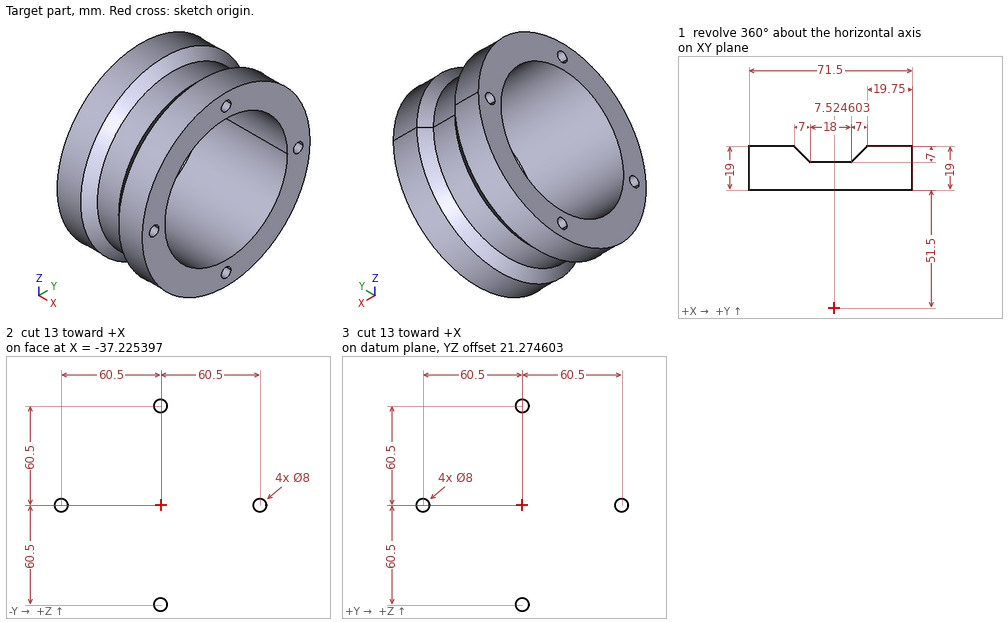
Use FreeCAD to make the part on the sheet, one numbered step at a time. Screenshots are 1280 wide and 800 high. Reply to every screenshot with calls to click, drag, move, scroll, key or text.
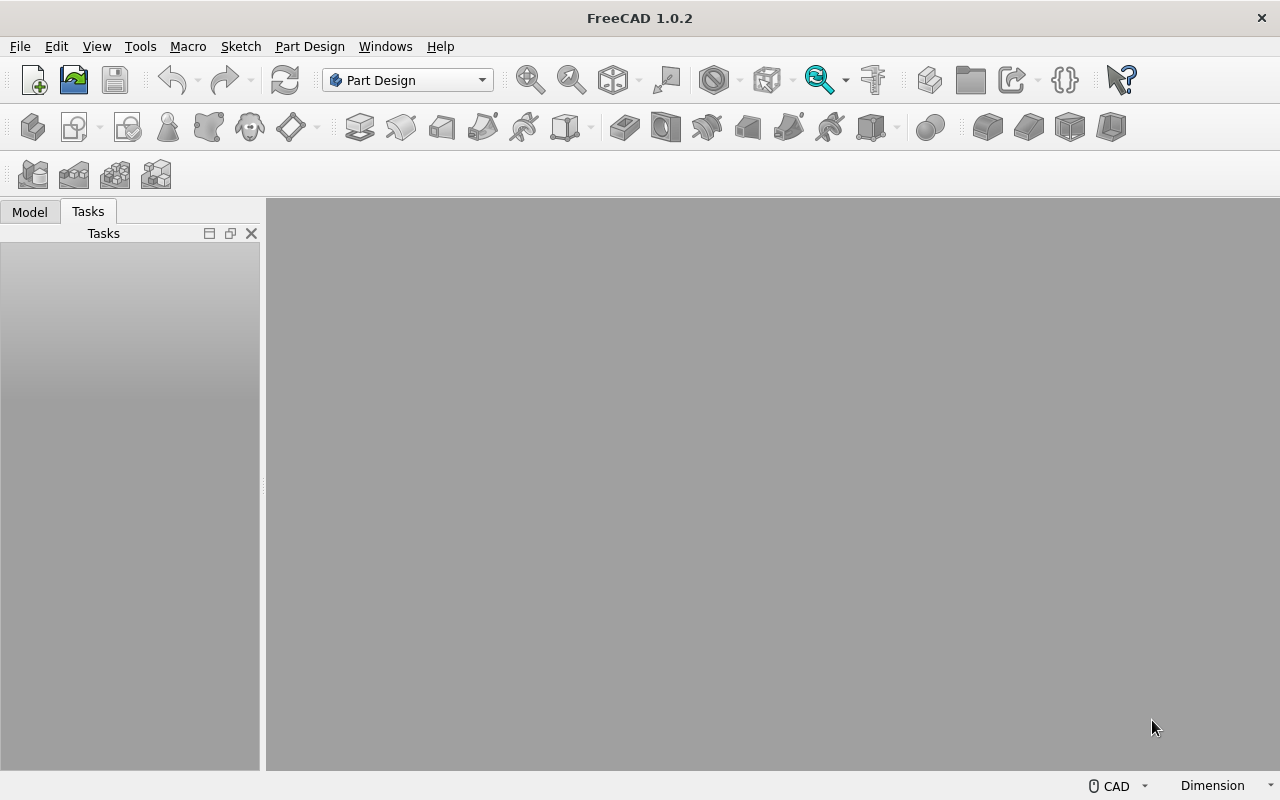
click(33, 80)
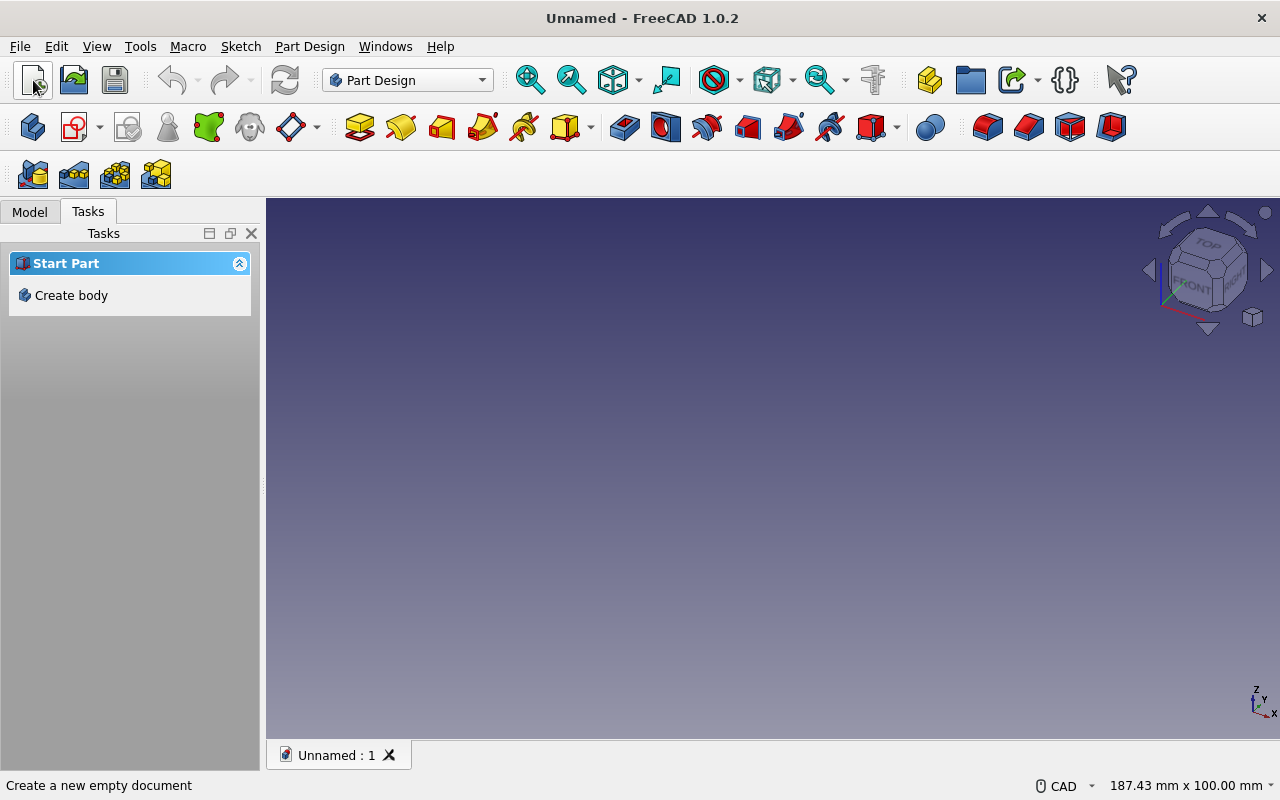
click(74, 128)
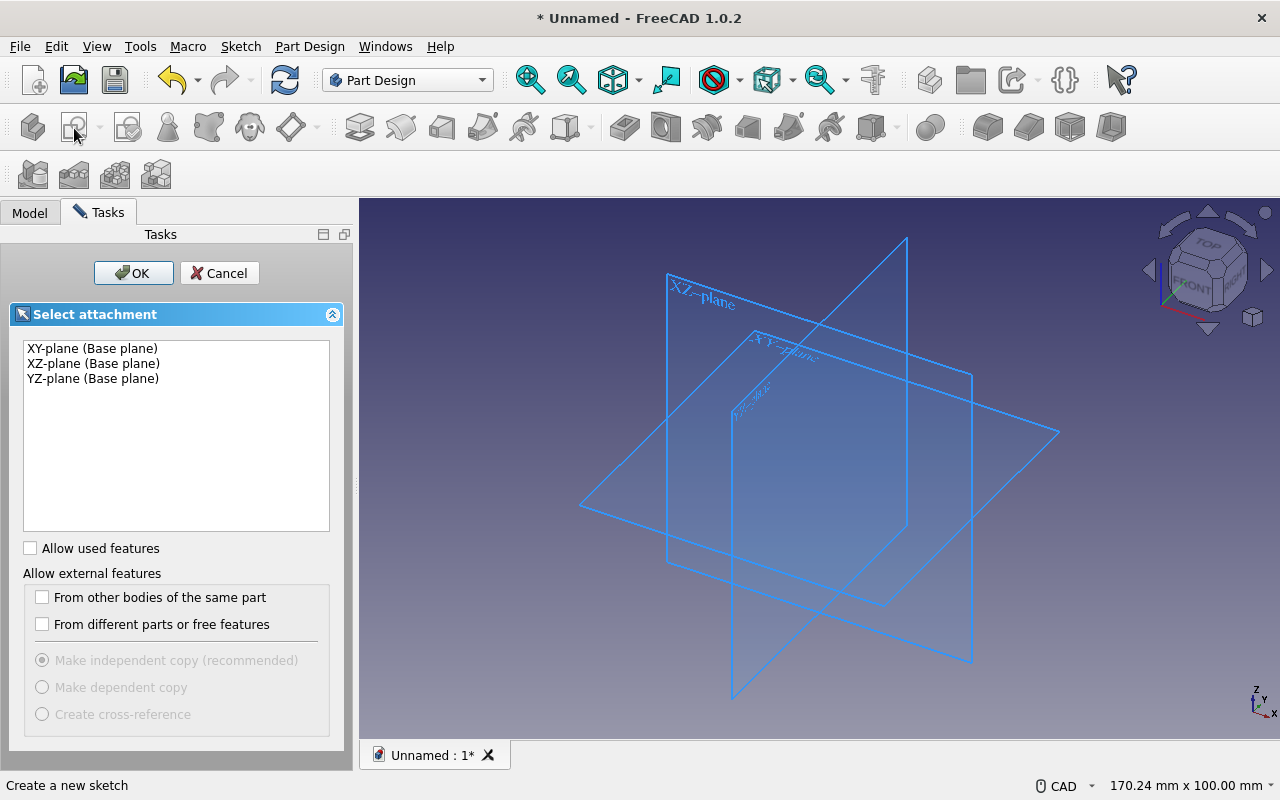
click(84, 348)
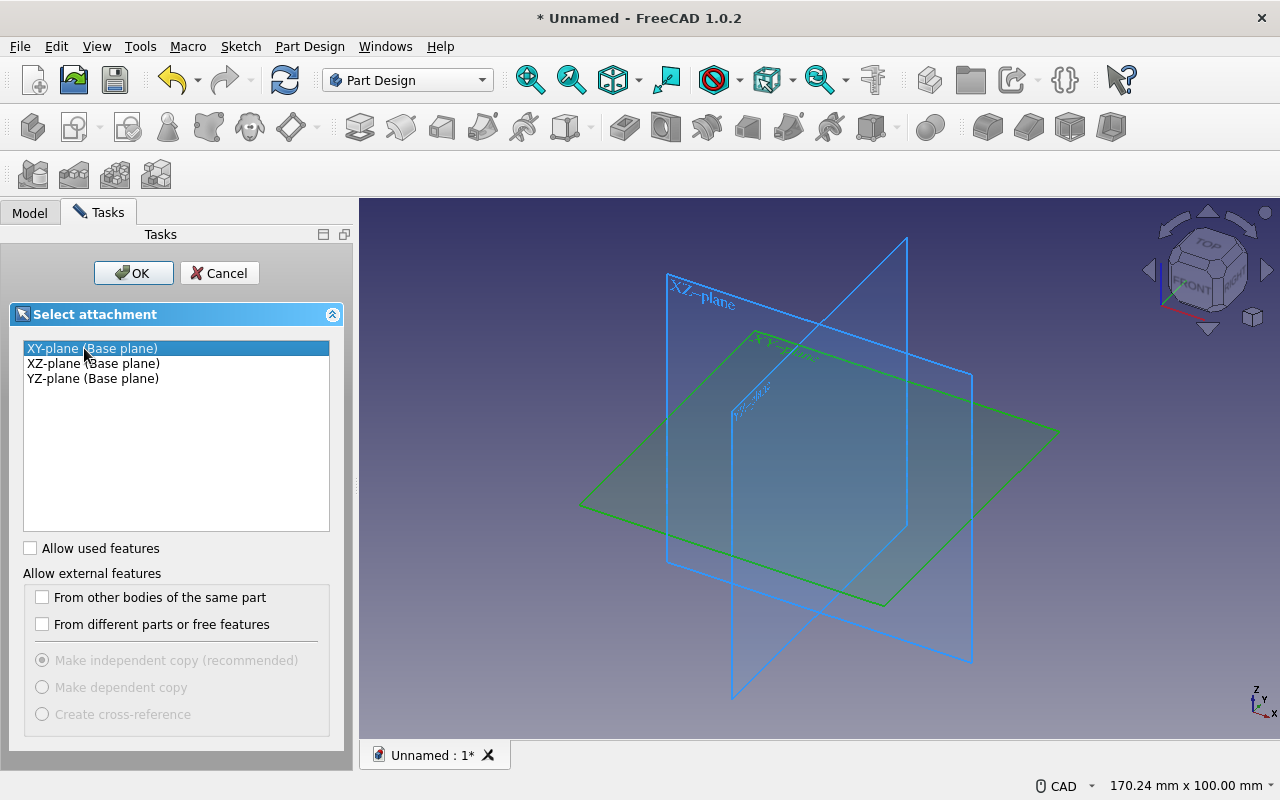
click(134, 273)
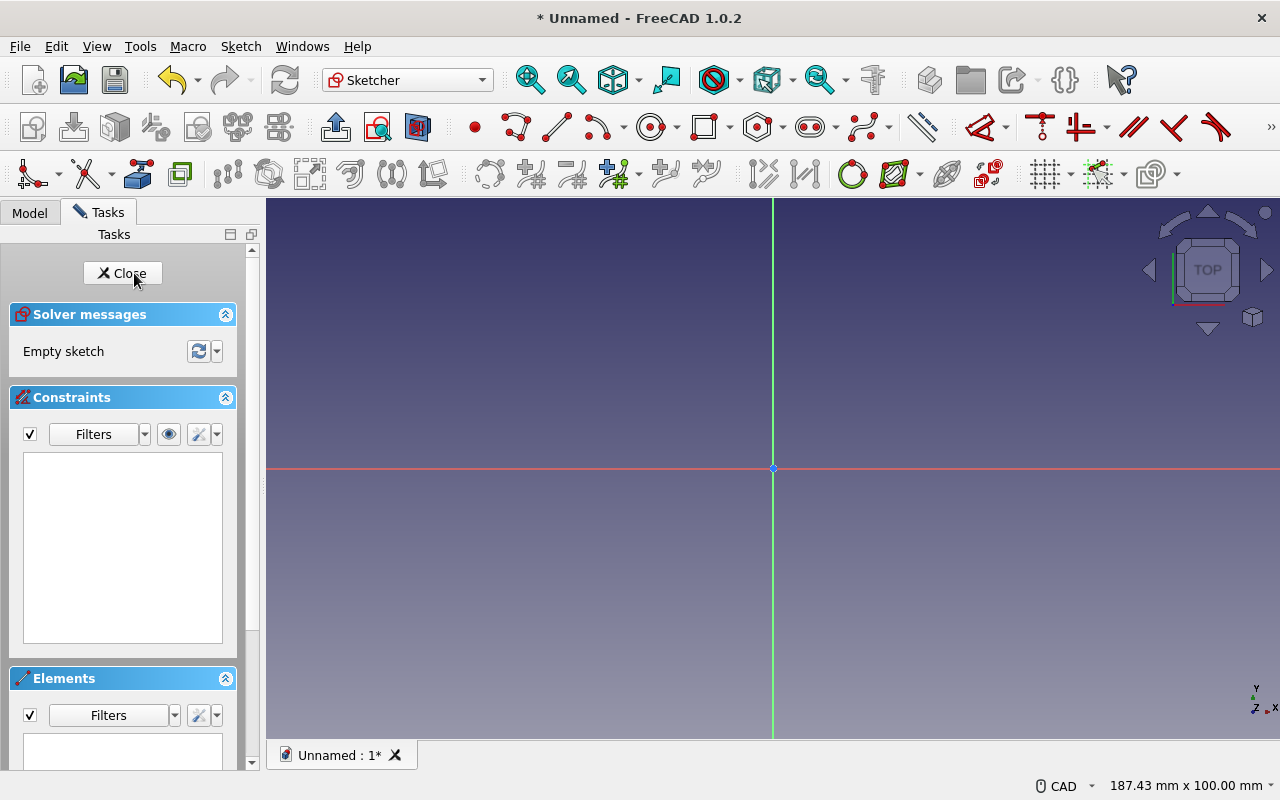
scroll(581, 711, down, 2)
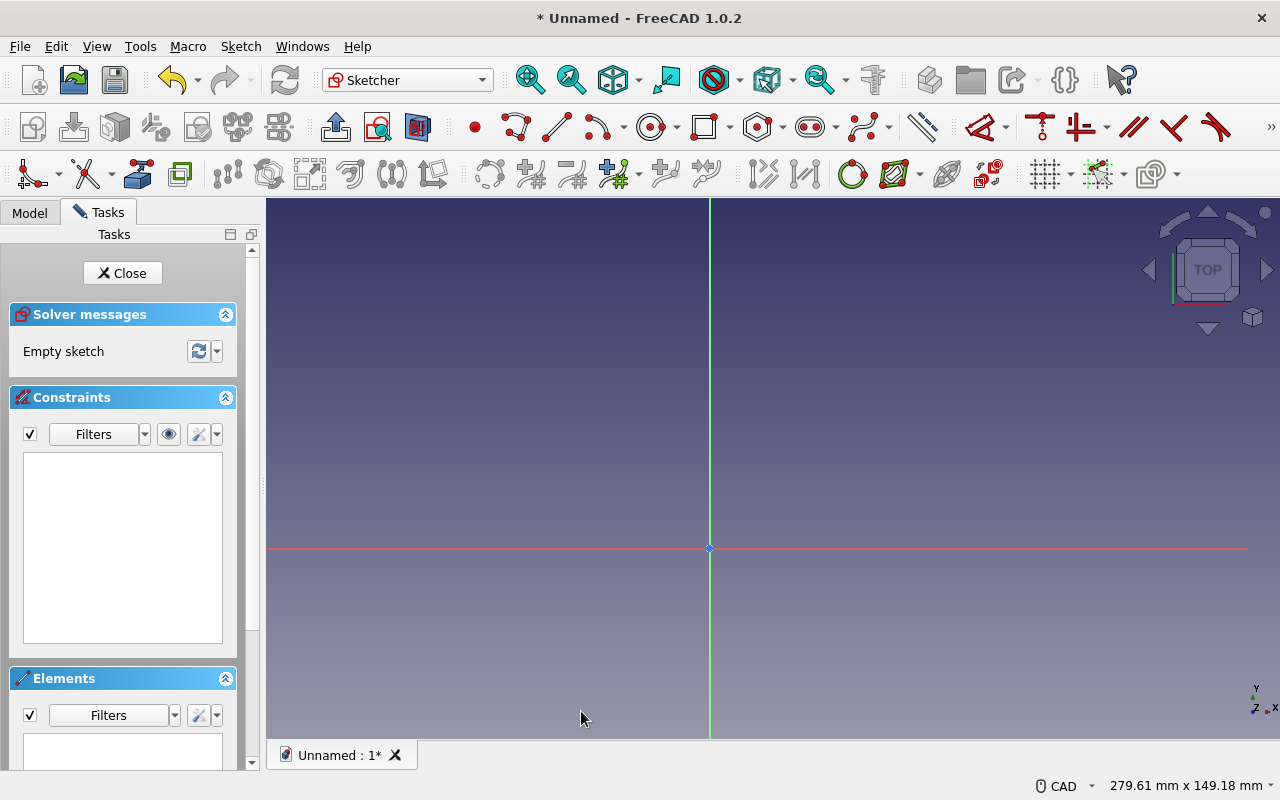
click(516, 128)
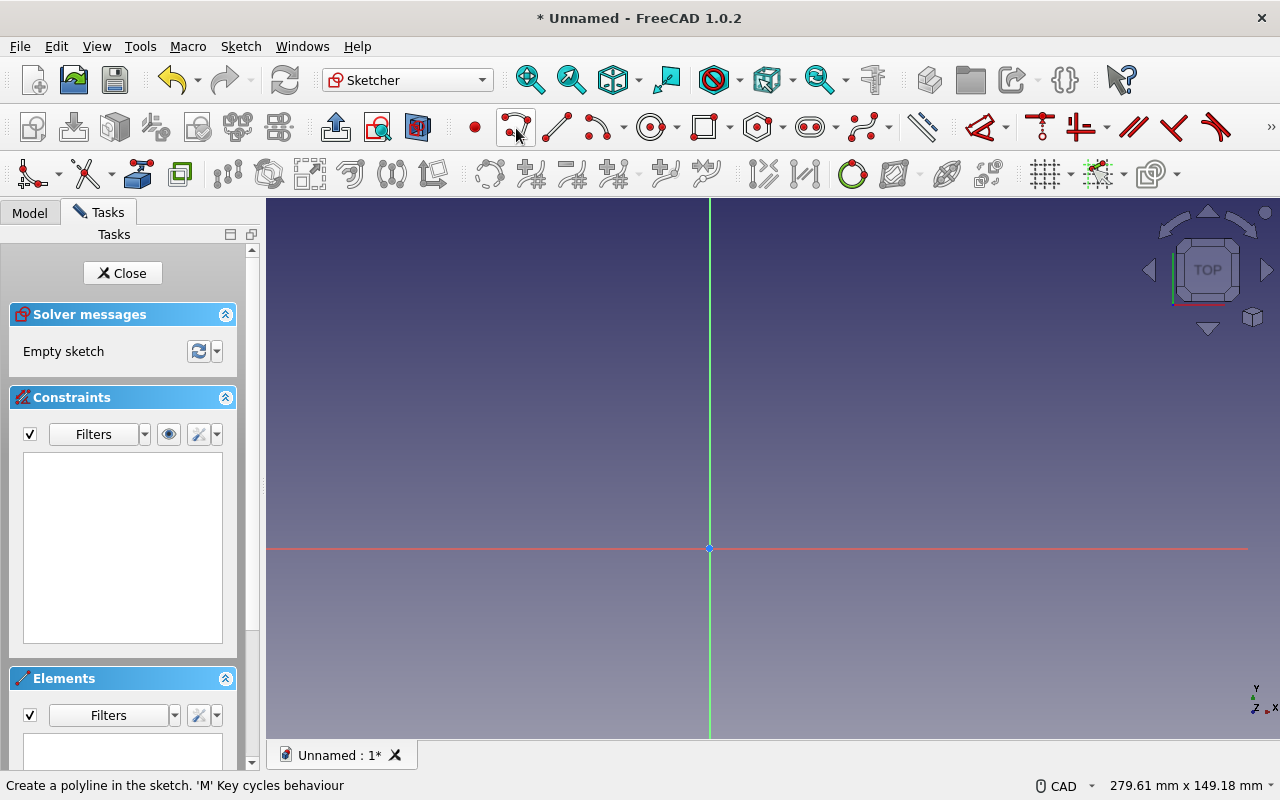
click(834, 362)
click(834, 293)
click(762, 293)
click(737, 318)
click(672, 318)
click(646, 293)
click(575, 293)
click(575, 362)
click(834, 363)
key(Escape)
key(Escape)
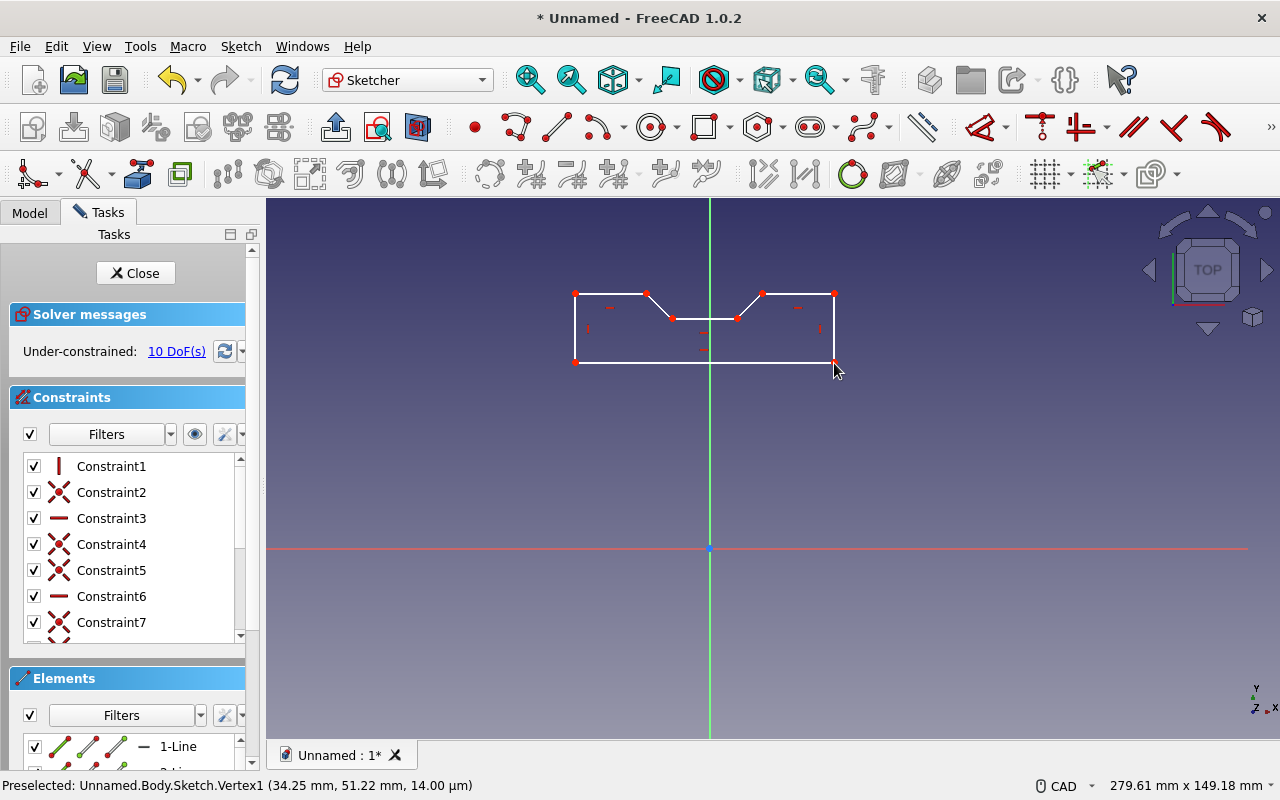
click(980, 128)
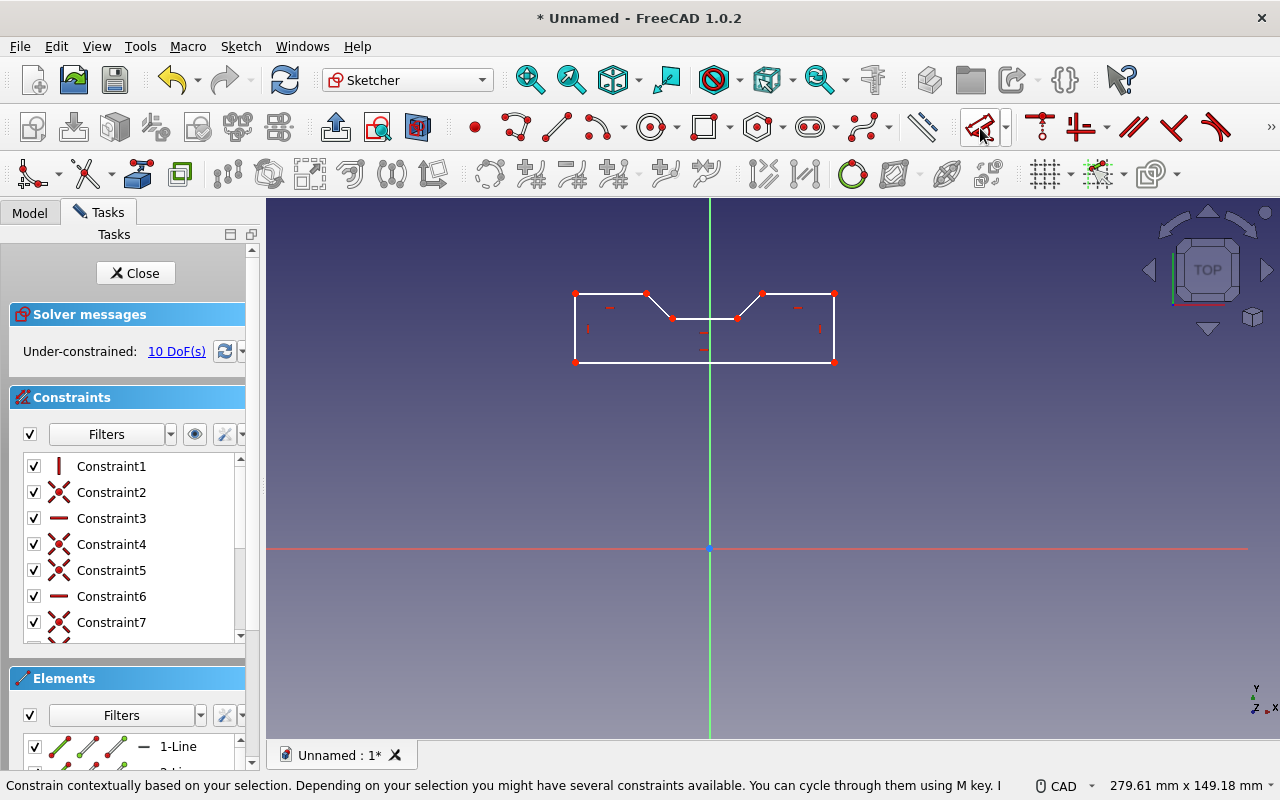
click(834, 342)
click(868, 328)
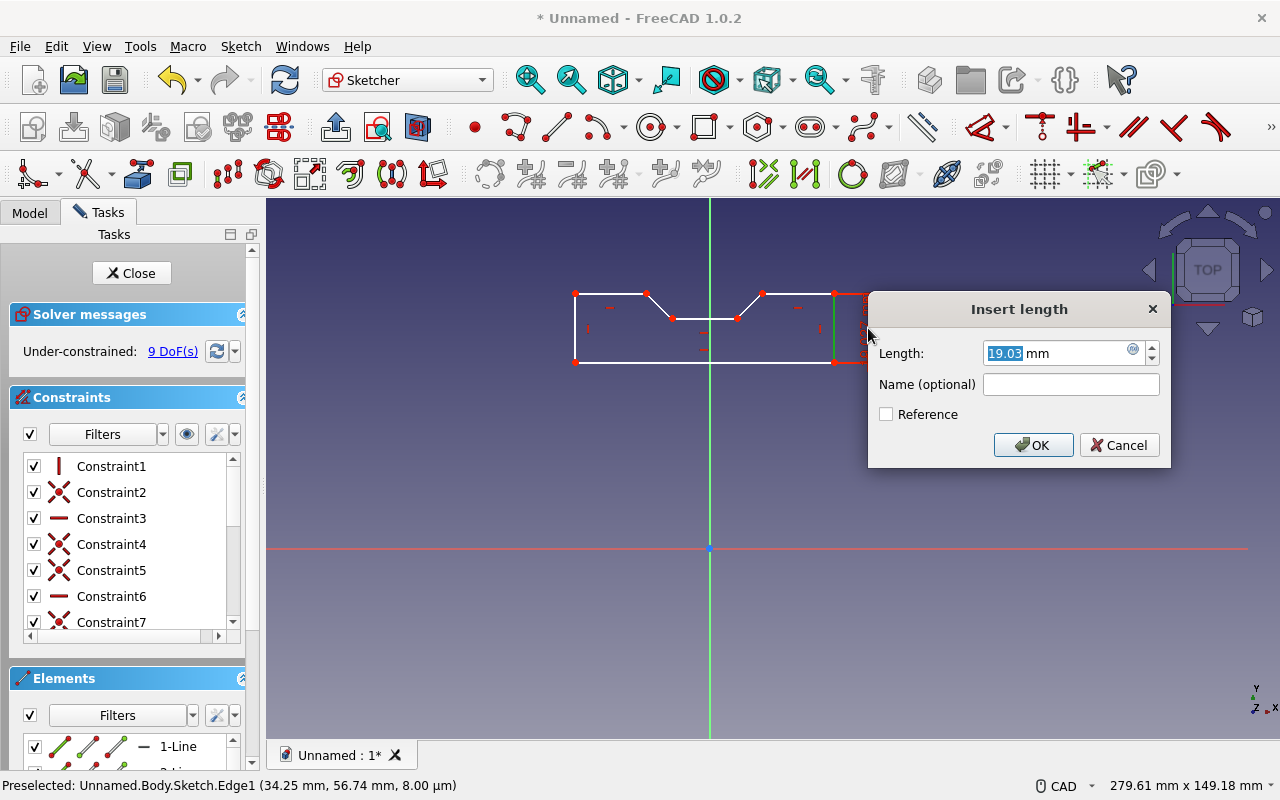
text(19)
key(Return)